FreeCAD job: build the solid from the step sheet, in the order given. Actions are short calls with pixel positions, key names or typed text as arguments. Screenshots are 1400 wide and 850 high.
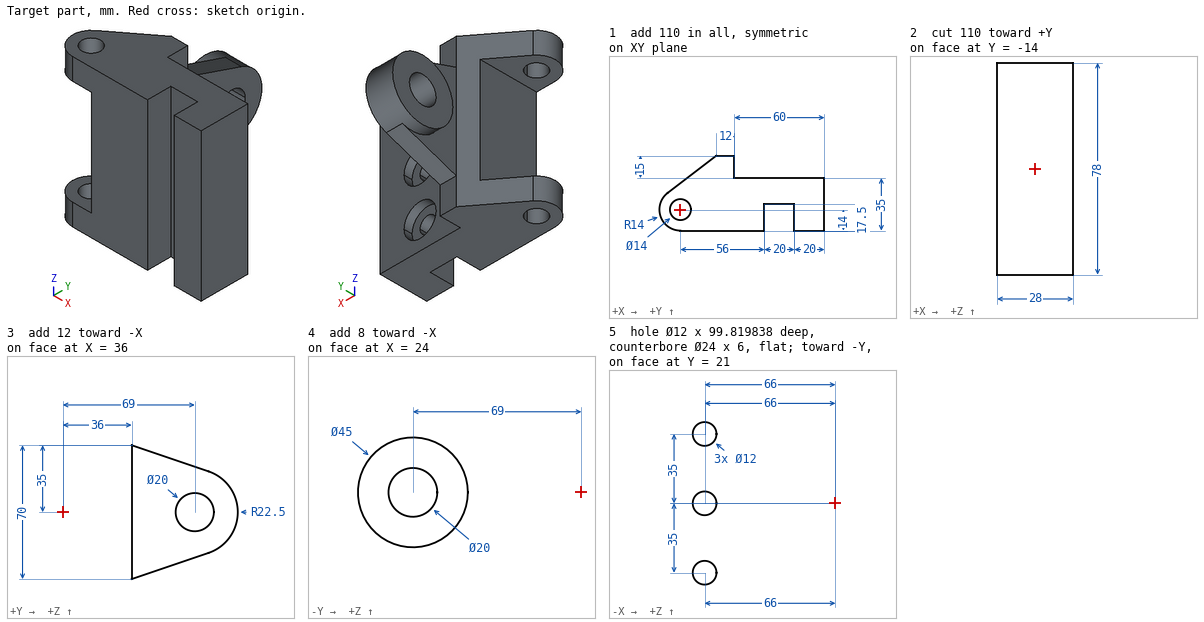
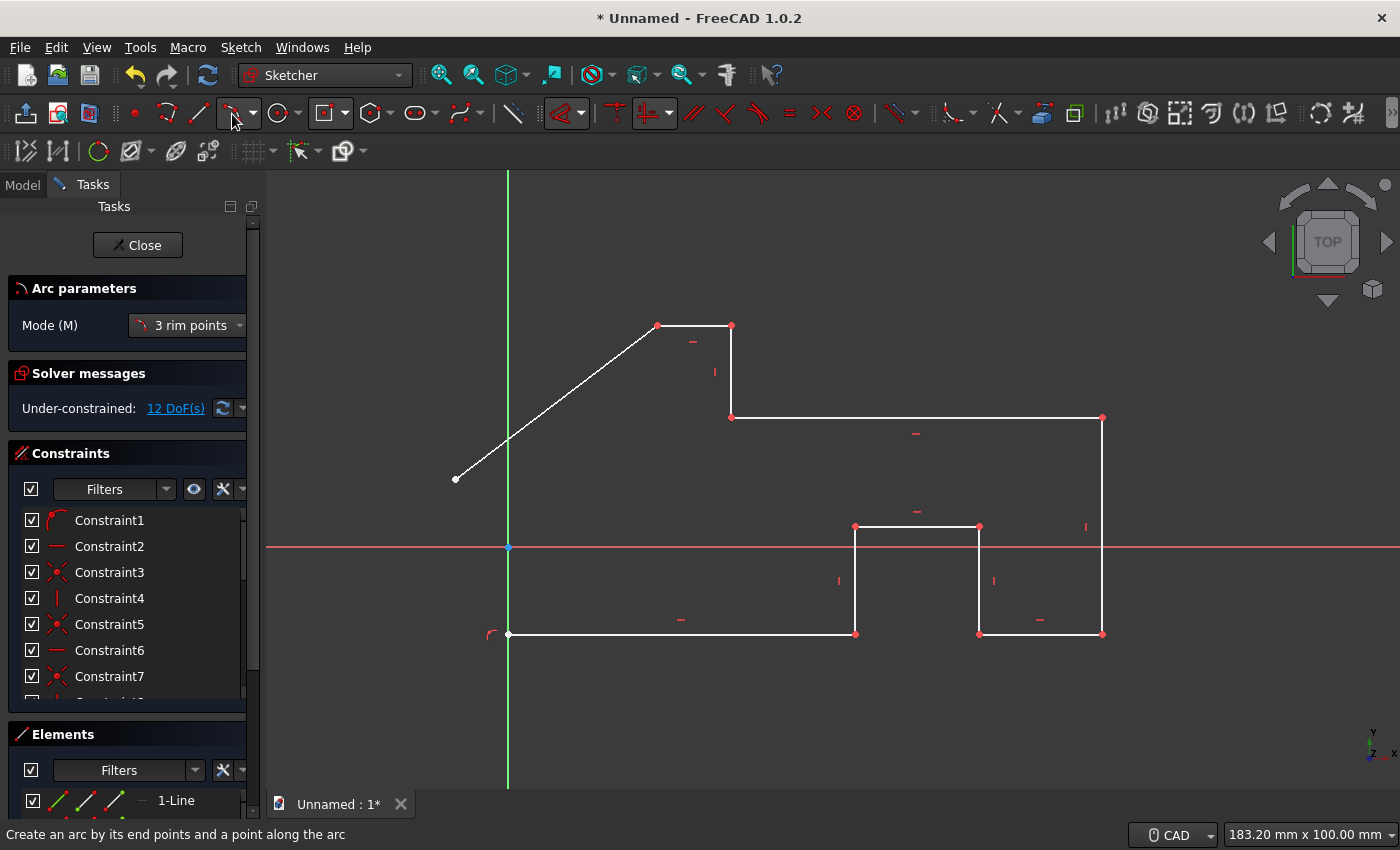
click(455, 480)
click(508, 635)
click(426, 575)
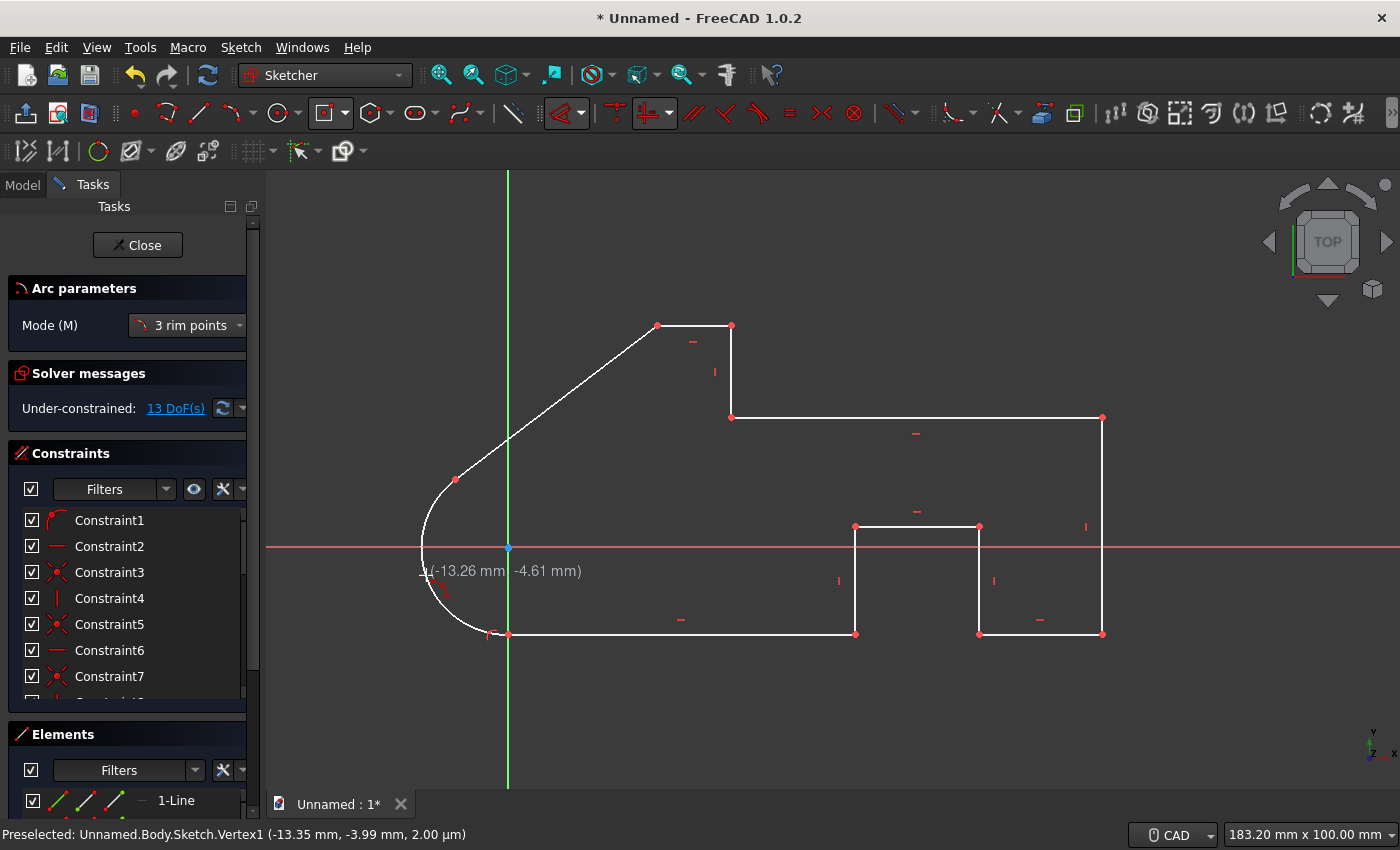
click(278, 114)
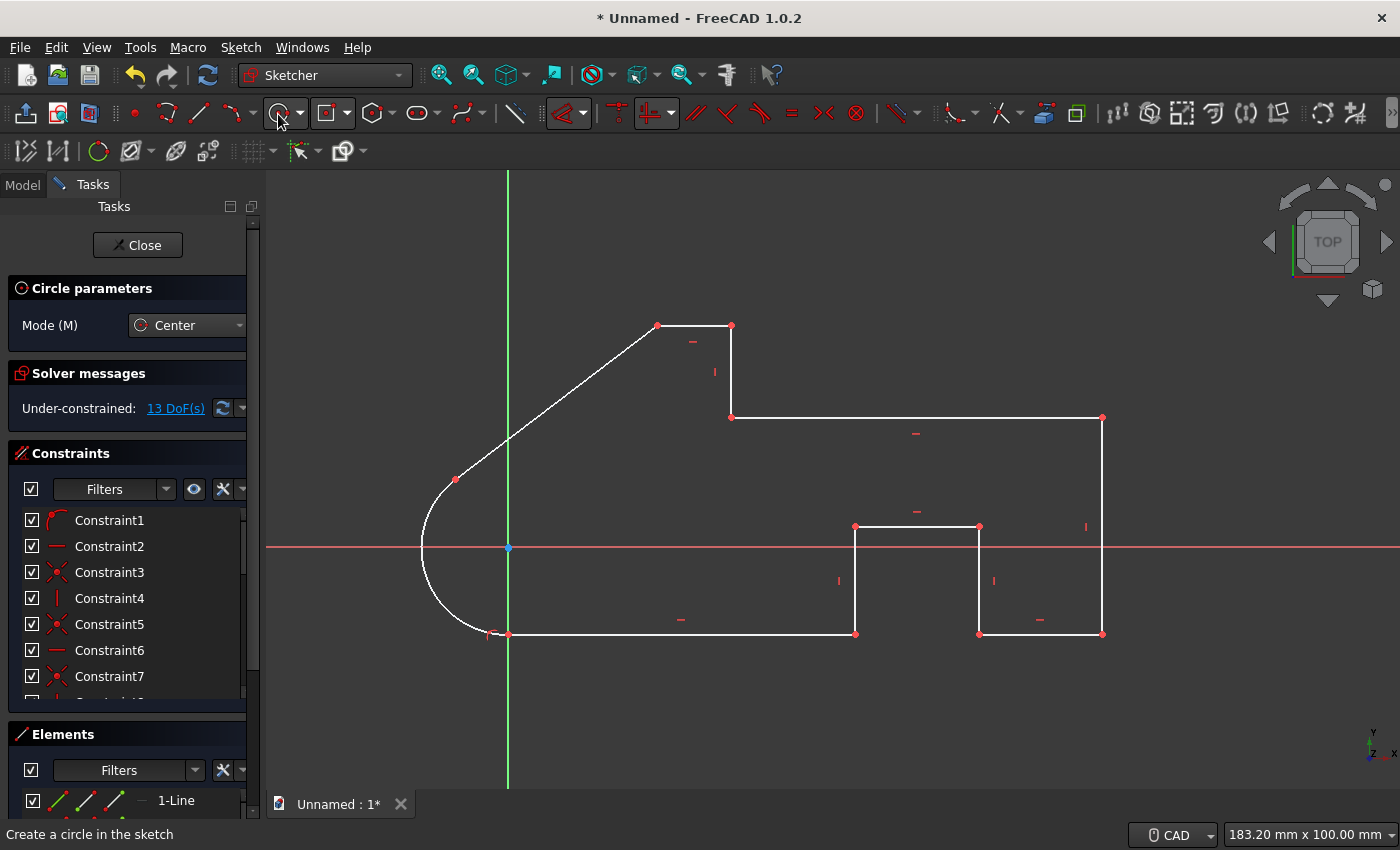
click(508, 547)
click(539, 517)
key(Escape)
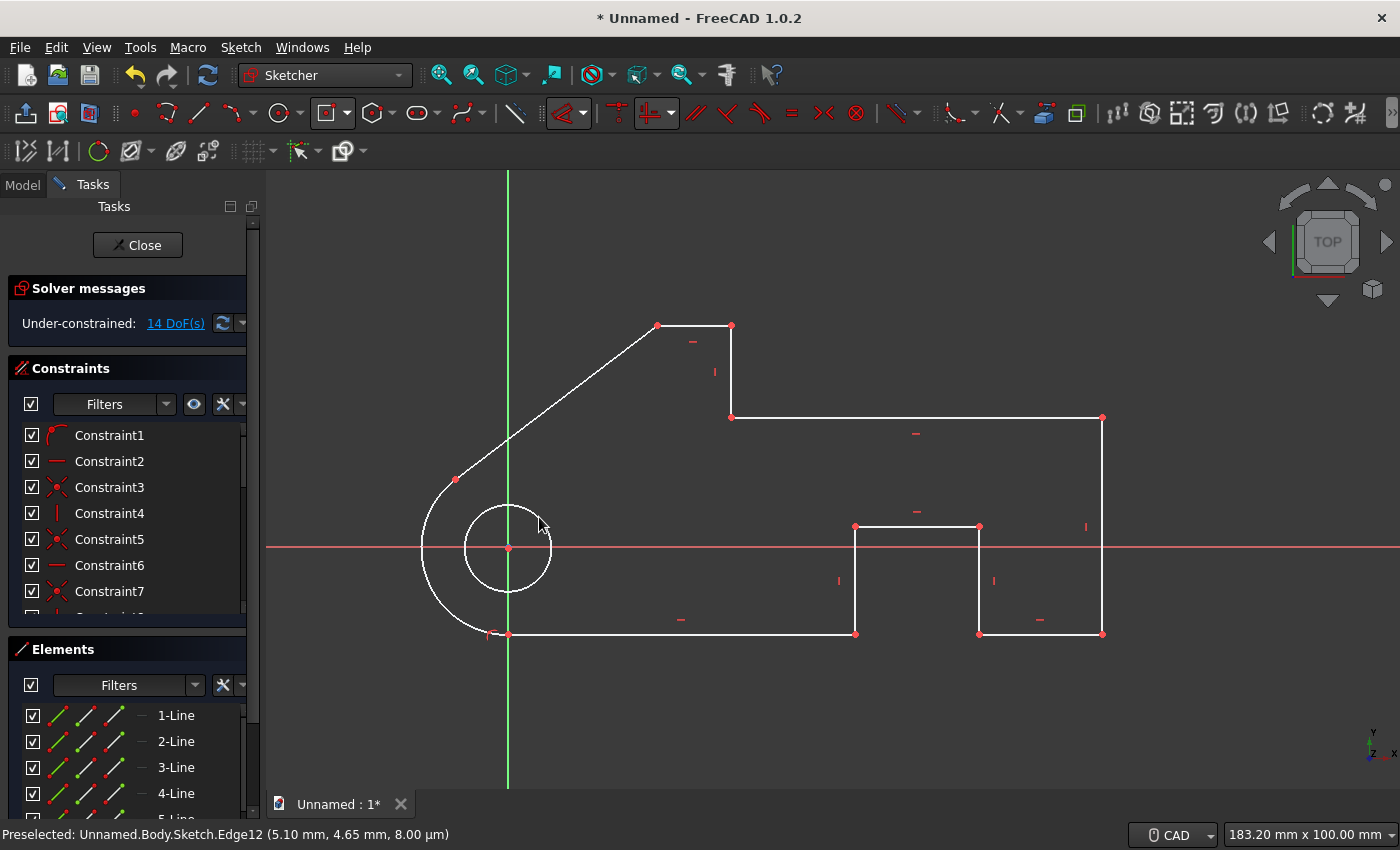
click(612, 635)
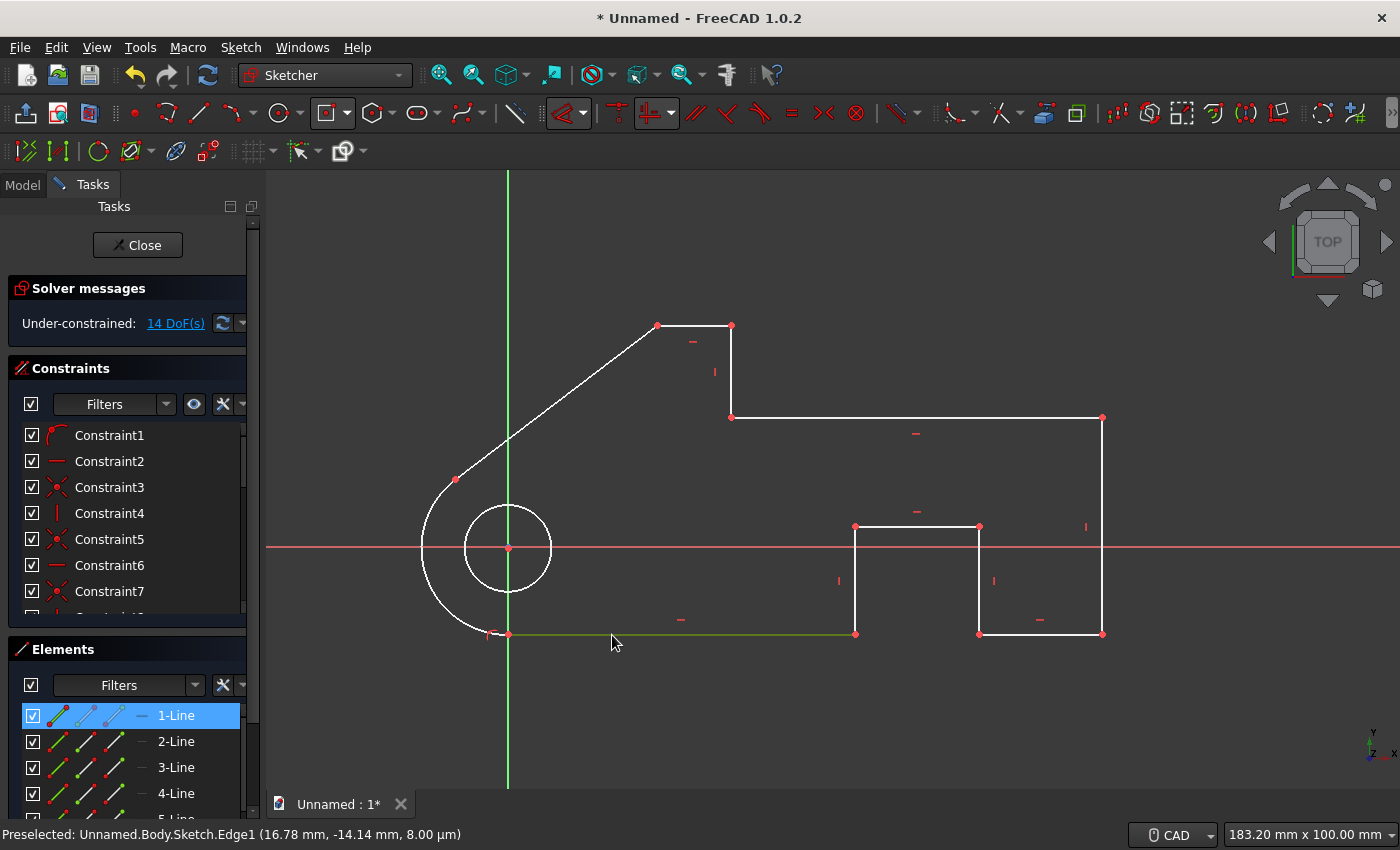
click(423, 534)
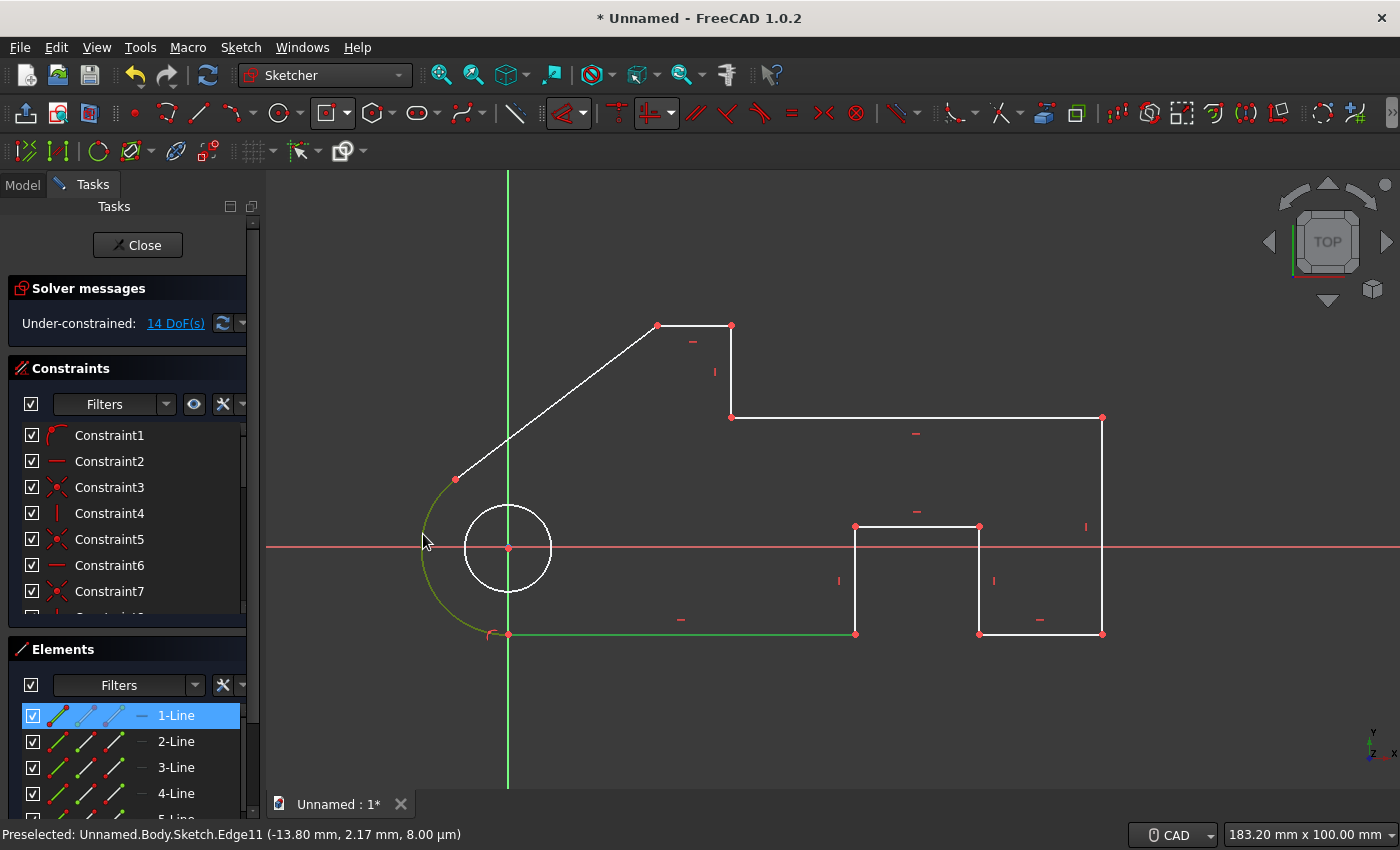
key(t)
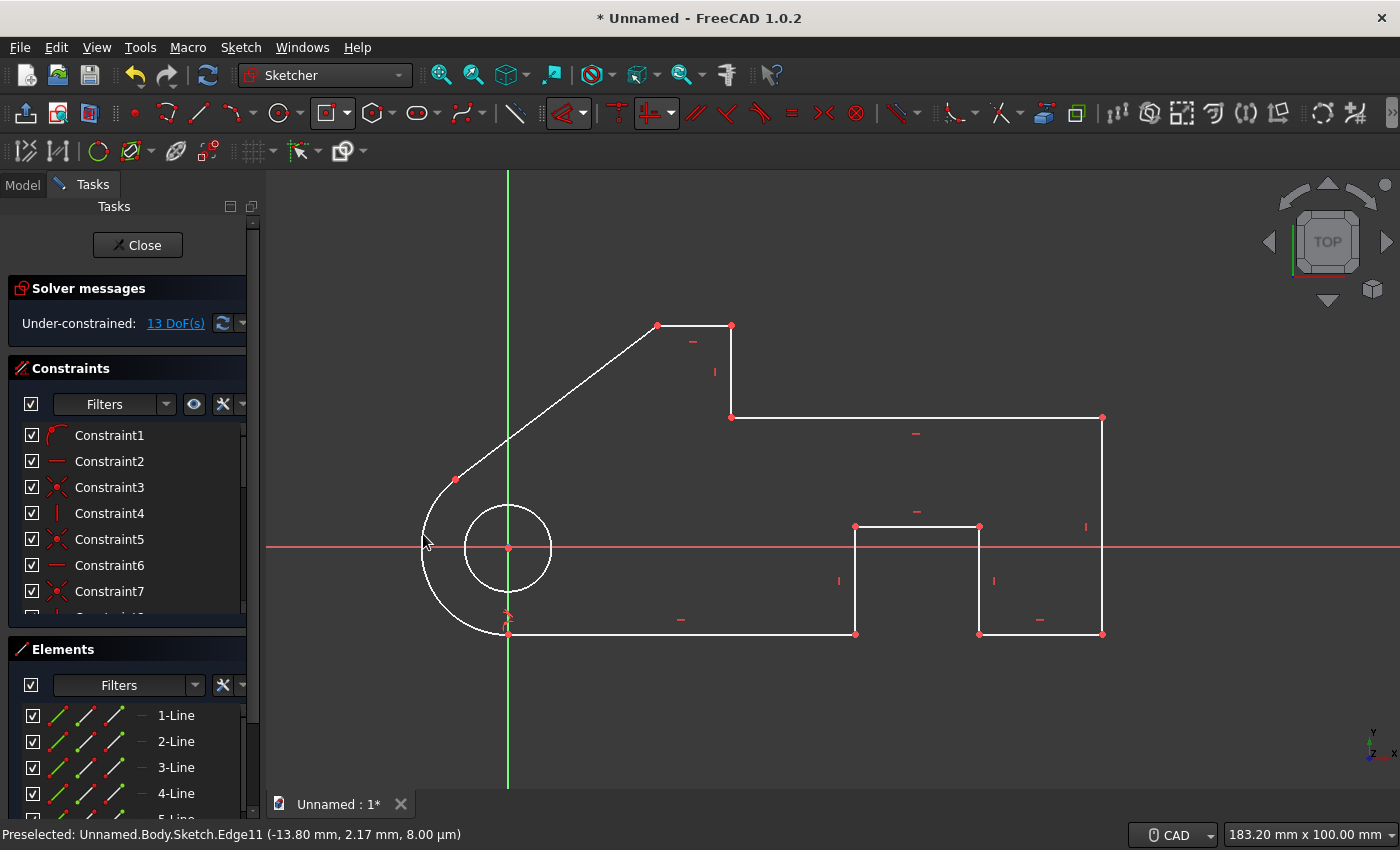
click(596, 372)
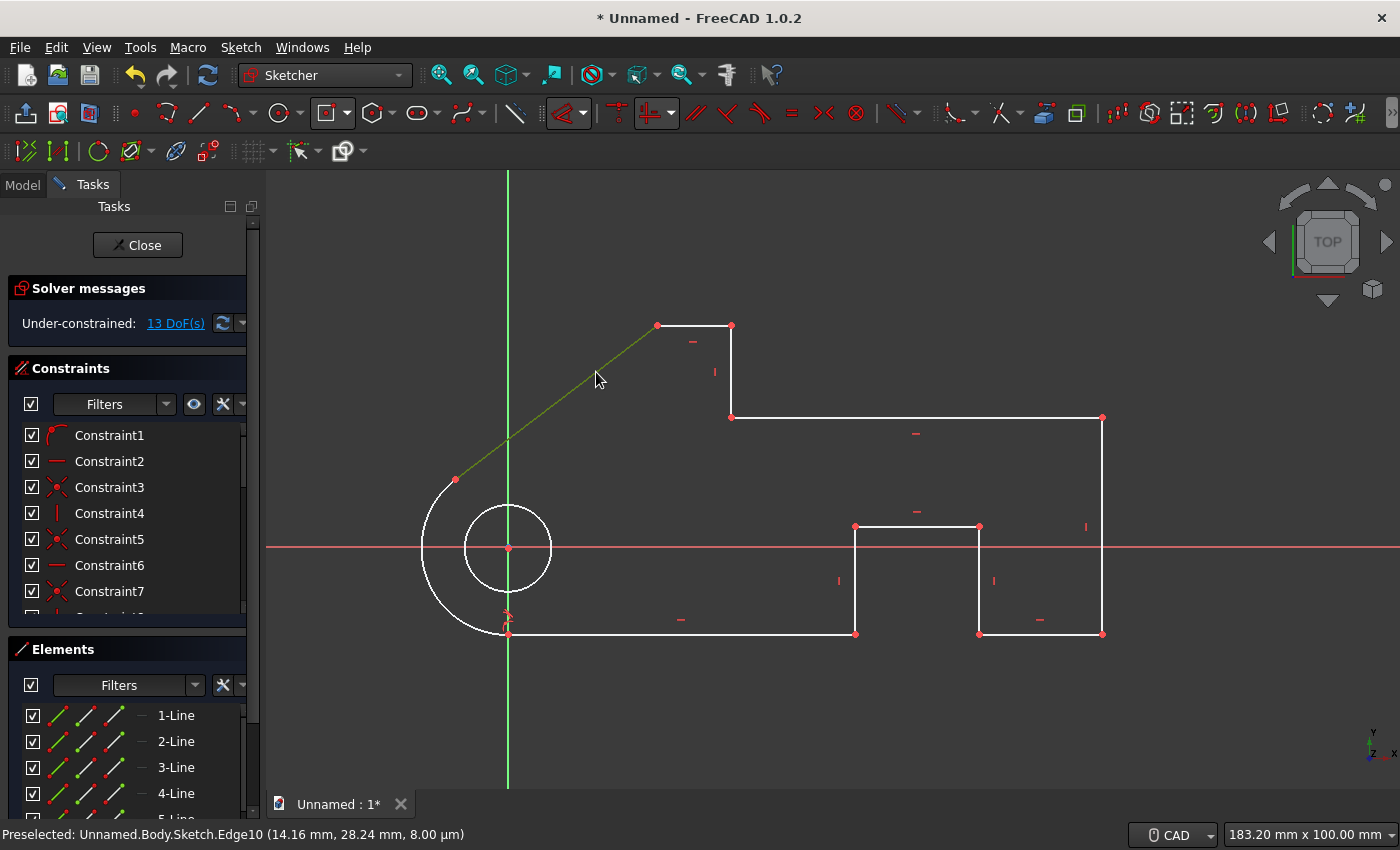
click(423, 534)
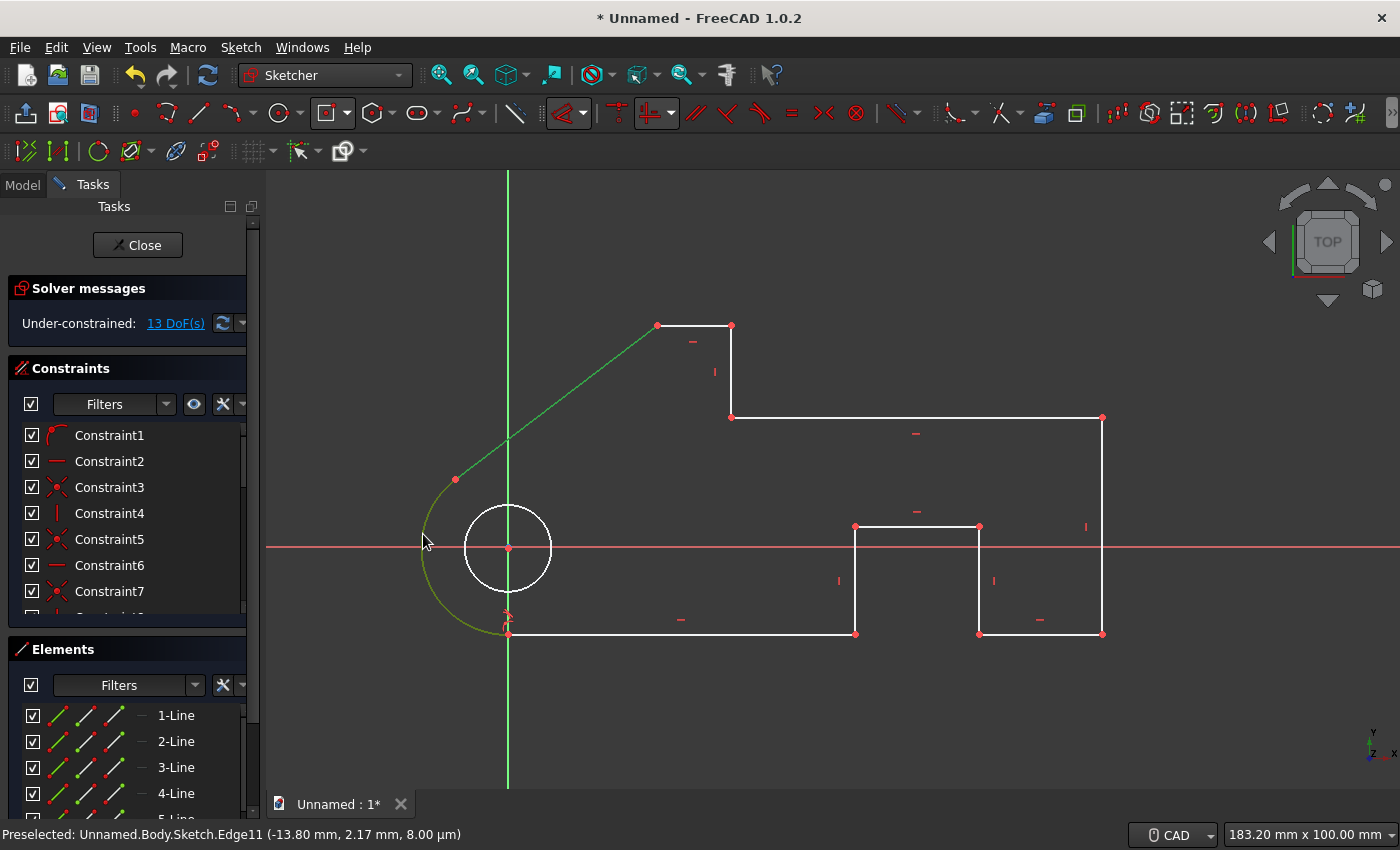
click(760, 114)